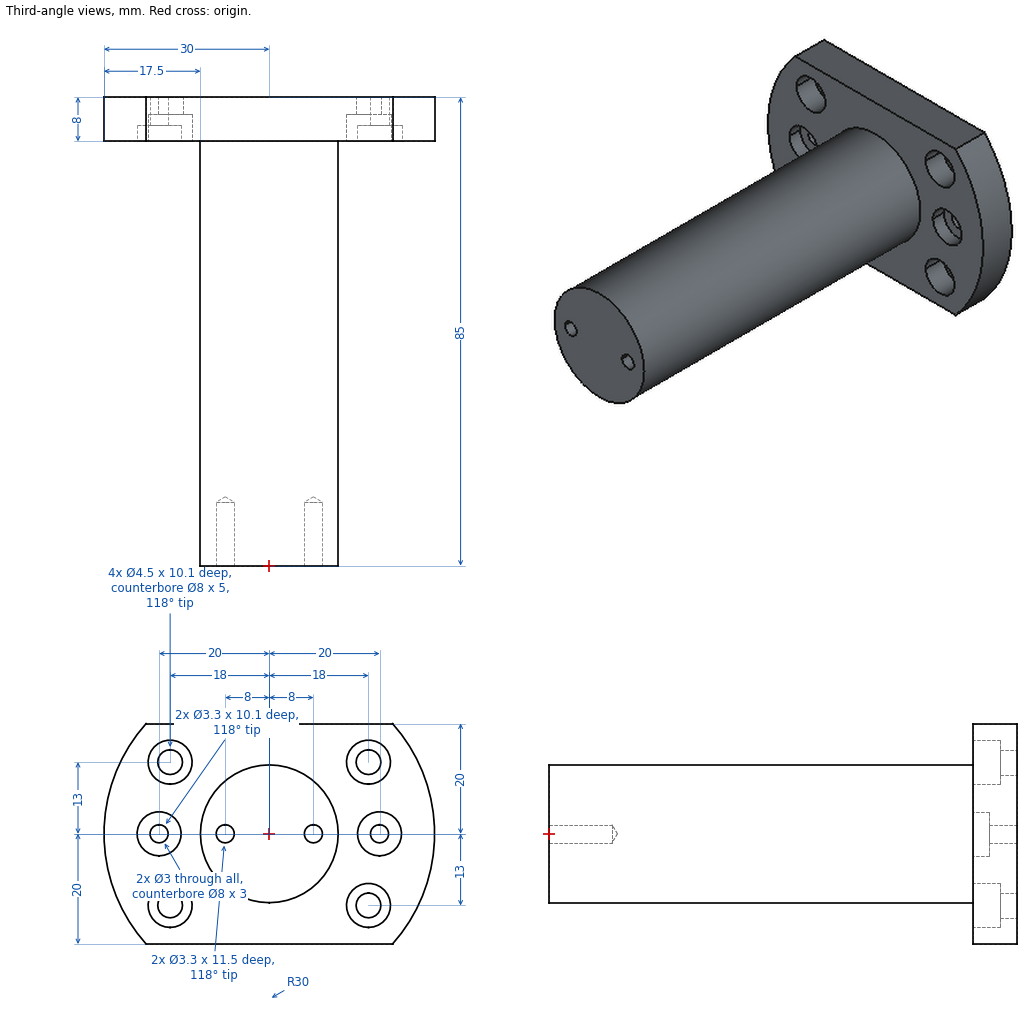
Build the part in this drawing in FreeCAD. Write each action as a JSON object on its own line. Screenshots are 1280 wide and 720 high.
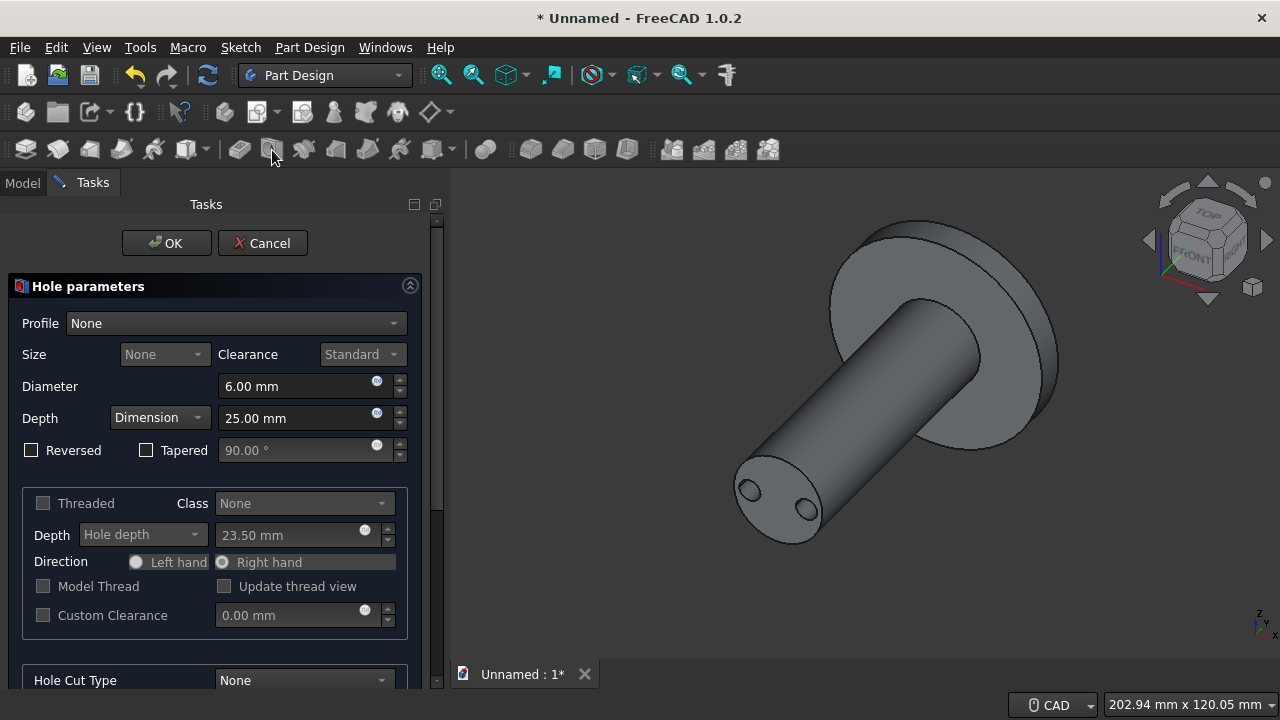
{"action": "triple_click", "coordinate": [305, 386]}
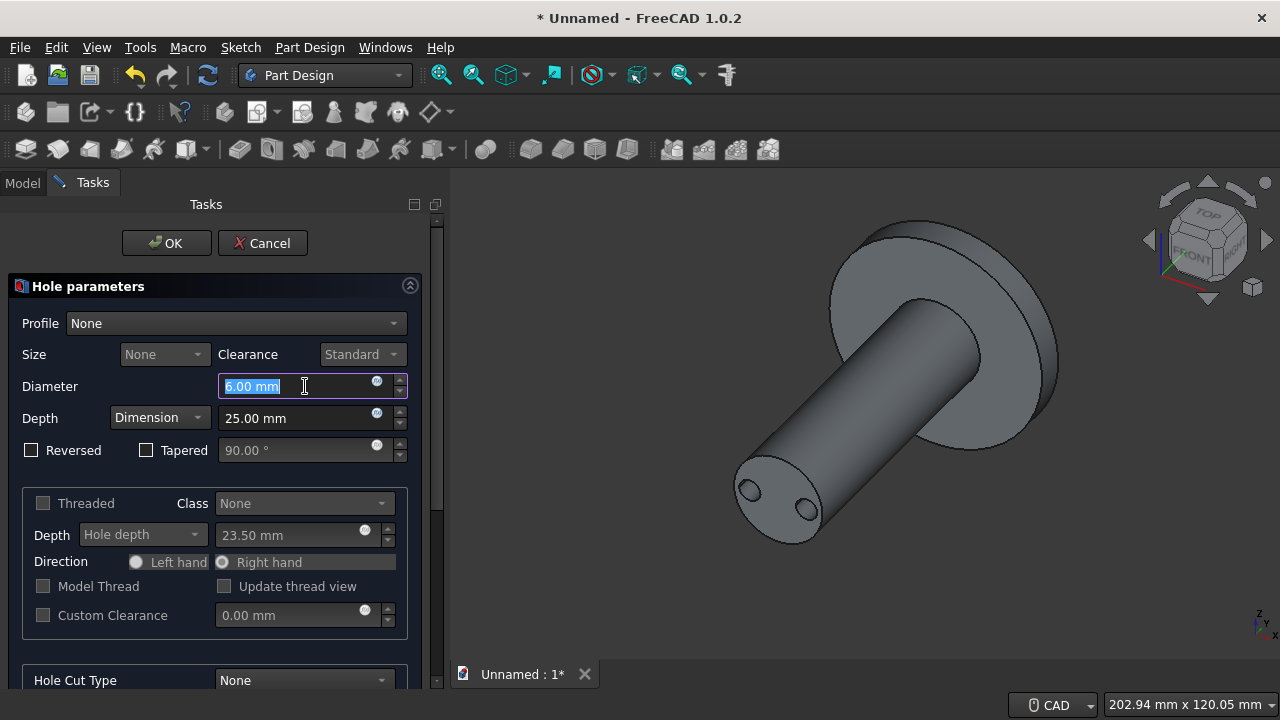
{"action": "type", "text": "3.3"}
{"action": "key", "text": "Tab"}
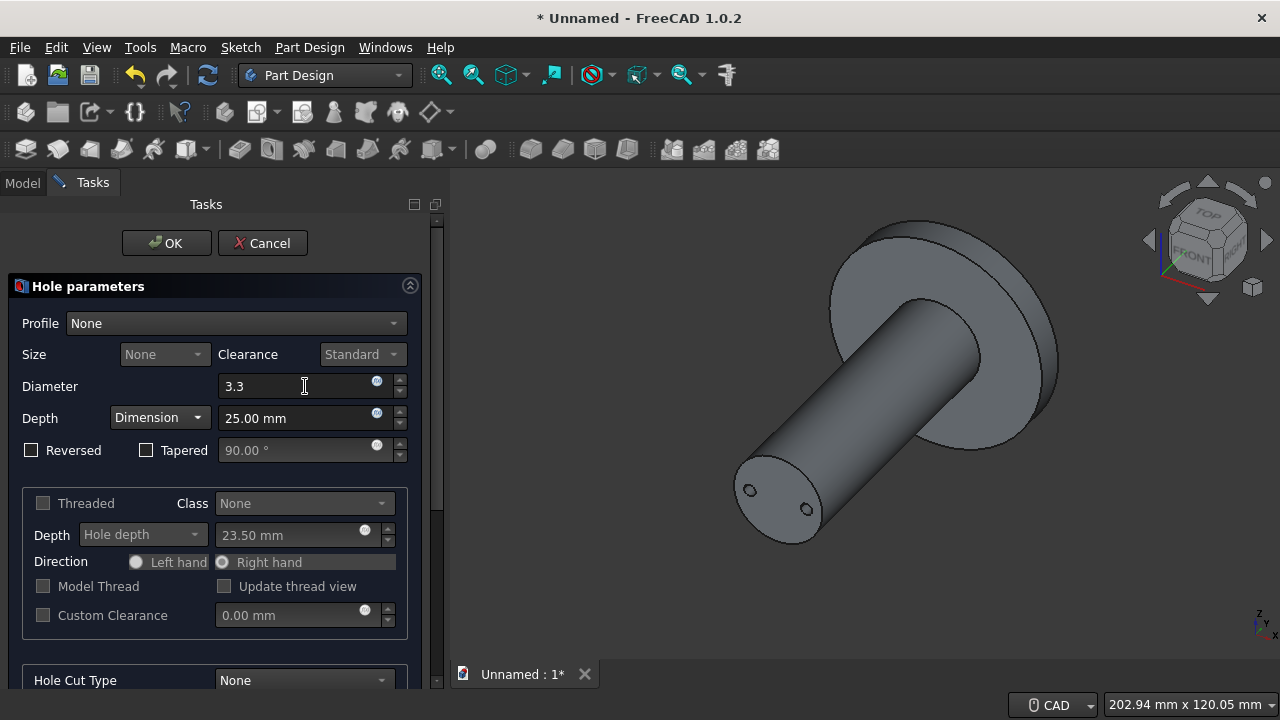
{"action": "triple_click", "coordinate": [305, 418]}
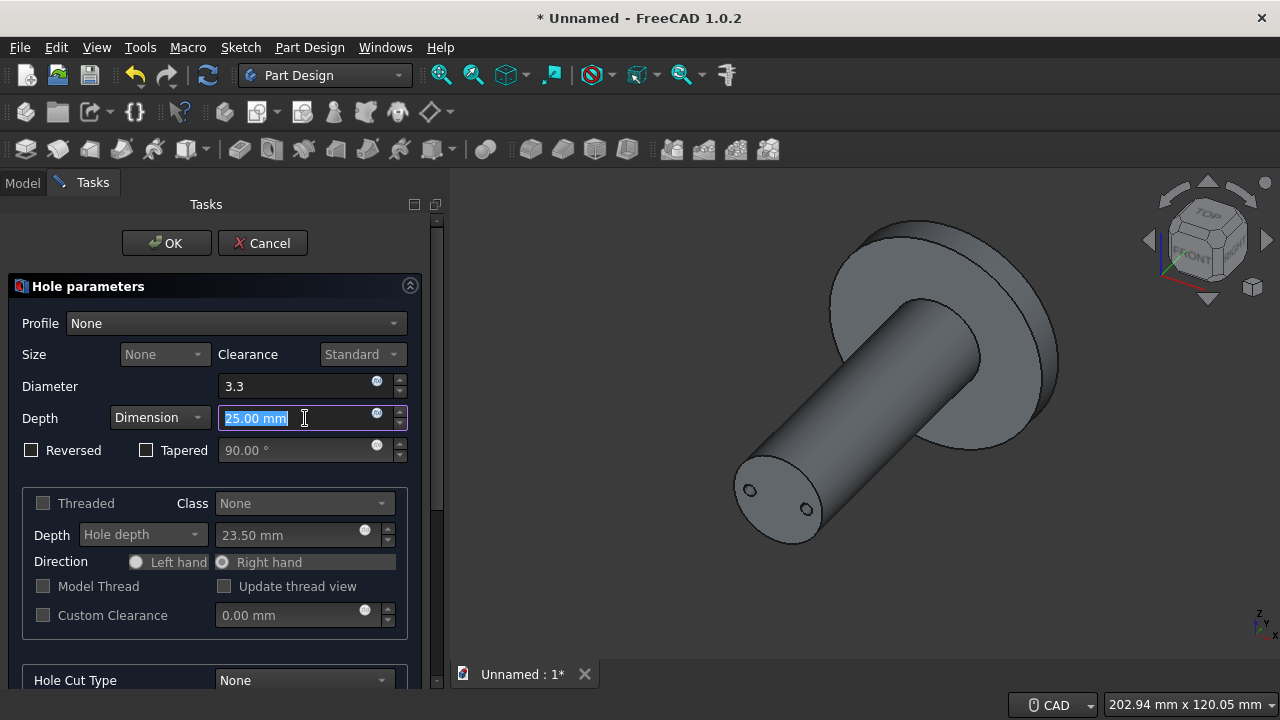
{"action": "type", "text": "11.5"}
{"action": "key", "text": "Tab"}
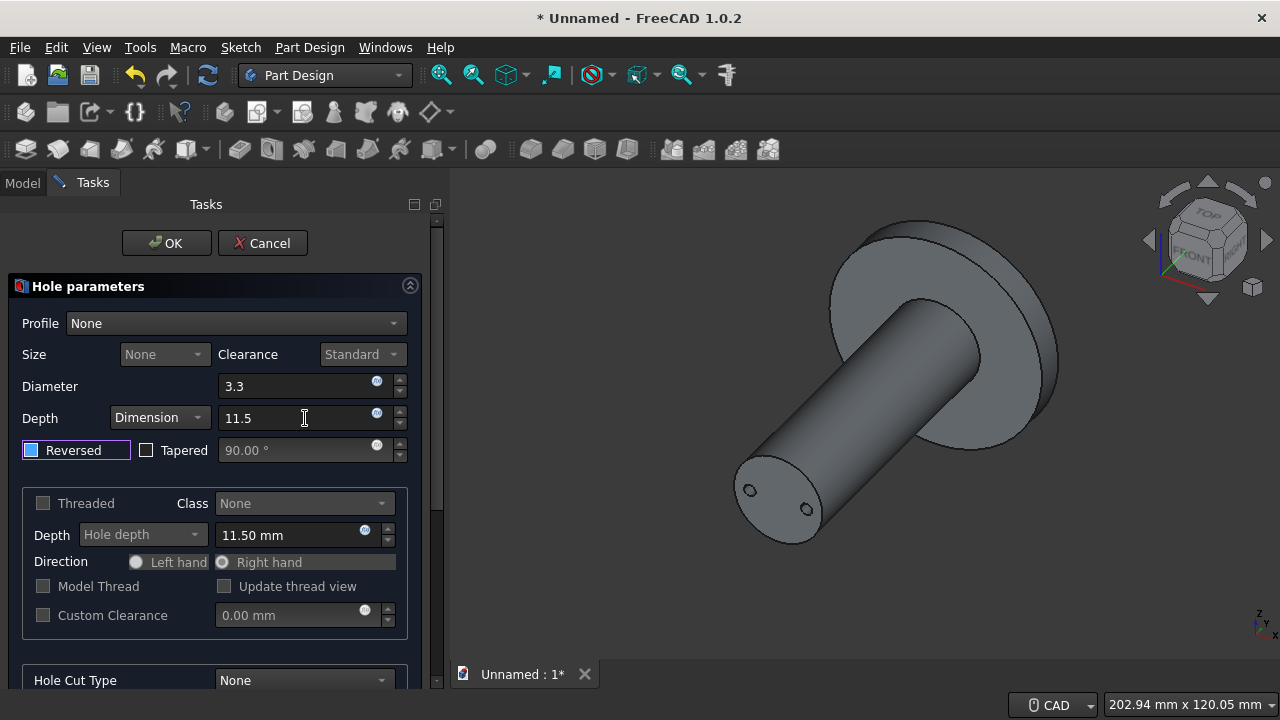
{"action": "left_click", "coordinate": [167, 243]}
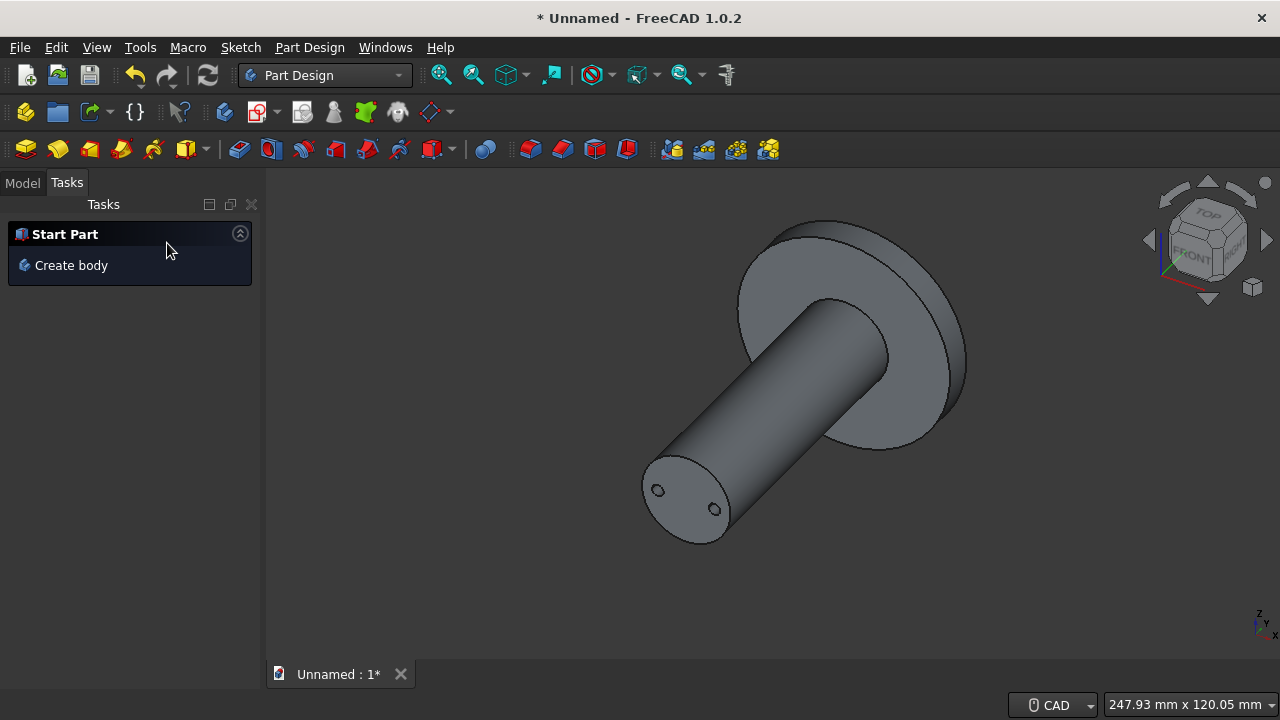
{"action": "key", "text": "4"}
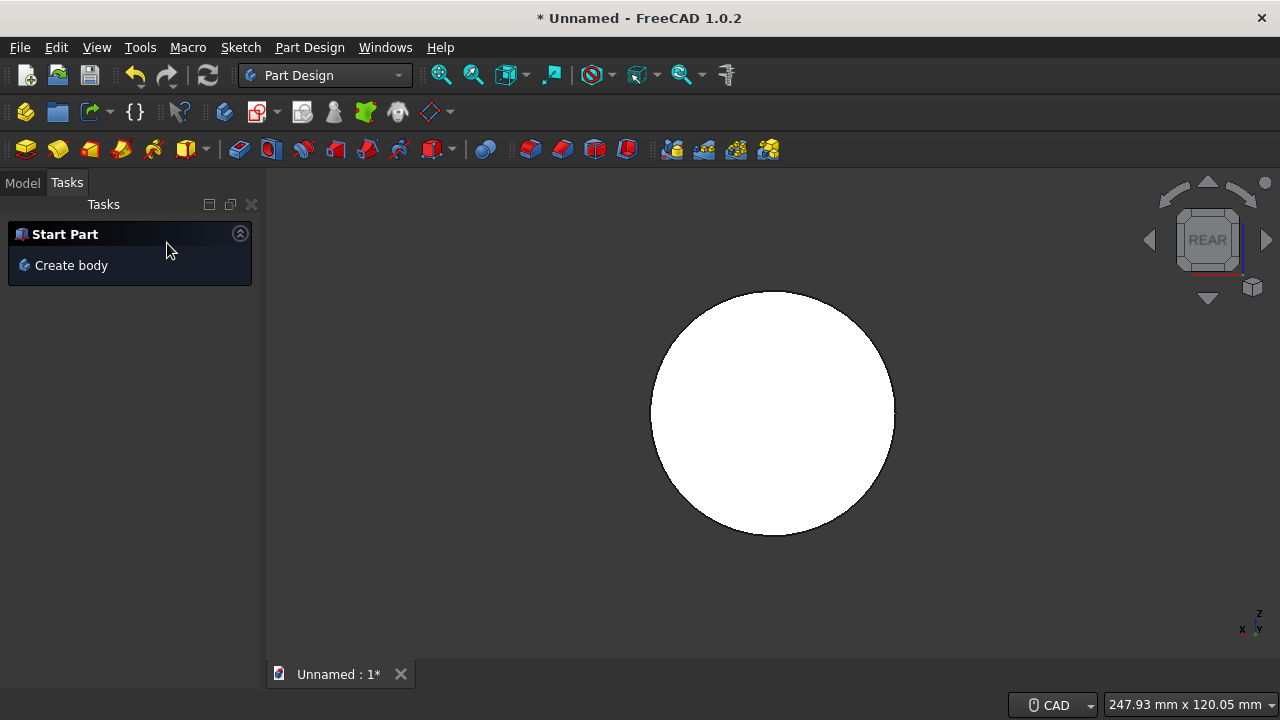
{"action": "left_click", "coordinate": [773, 412]}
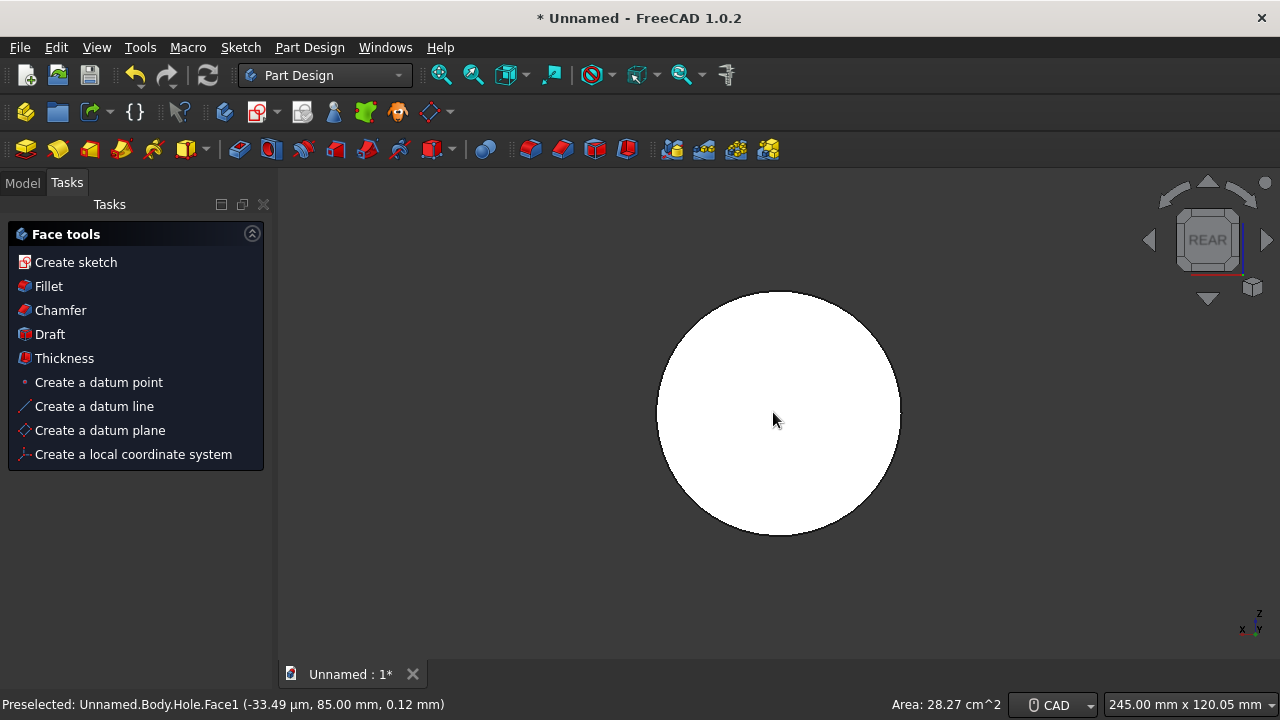
{"action": "left_click", "coordinate": [258, 112]}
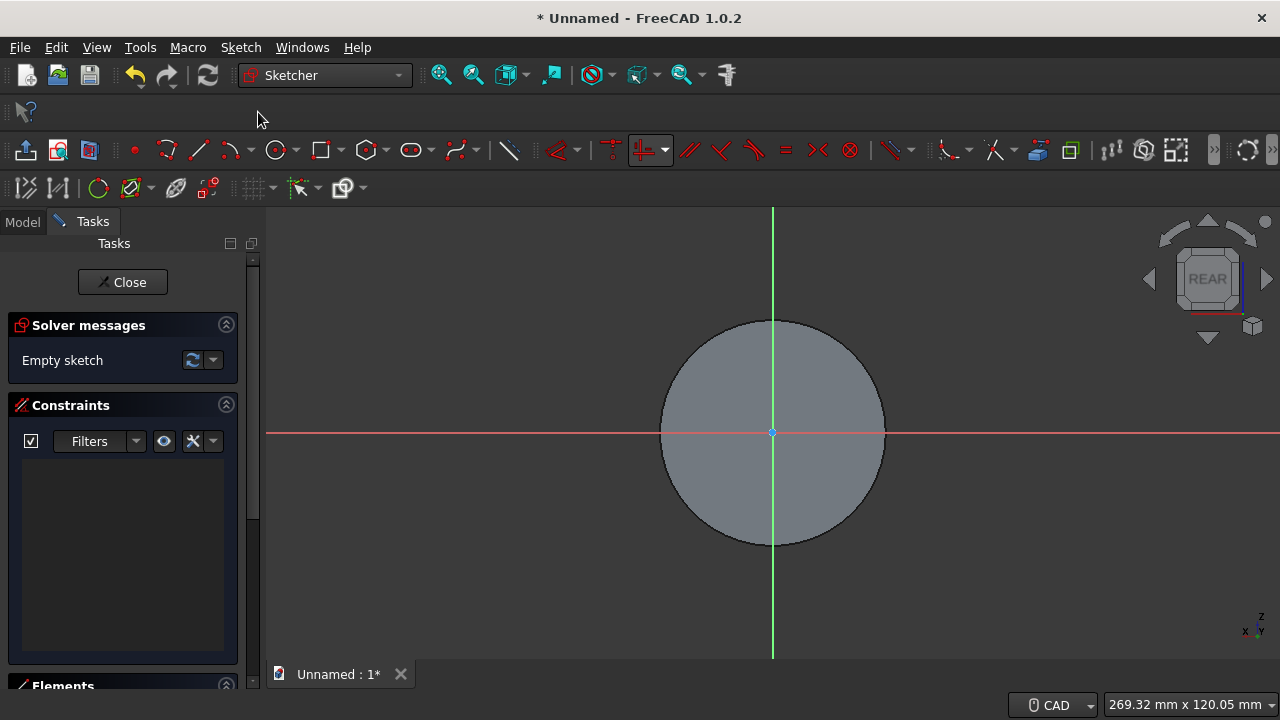
{"action": "scroll", "coordinate": [813, 522], "scroll_direction": "up", "scroll_amount": 5}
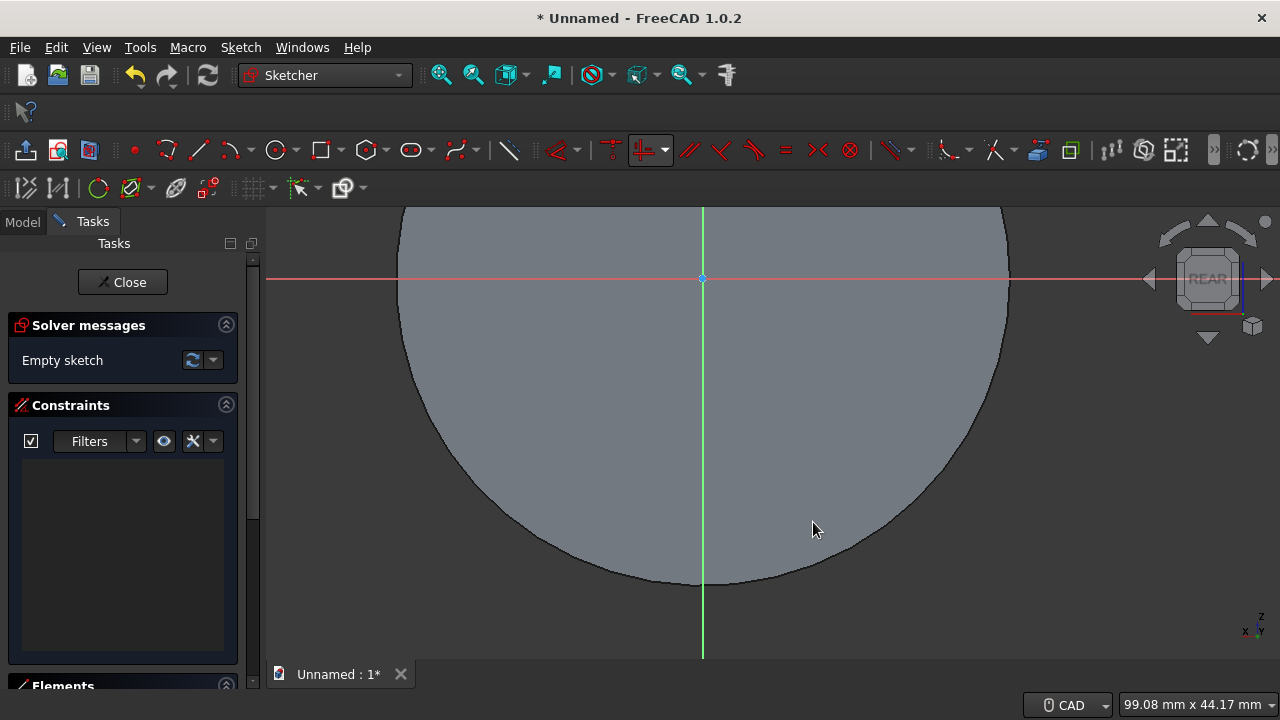
{"action": "left_click", "coordinate": [200, 150]}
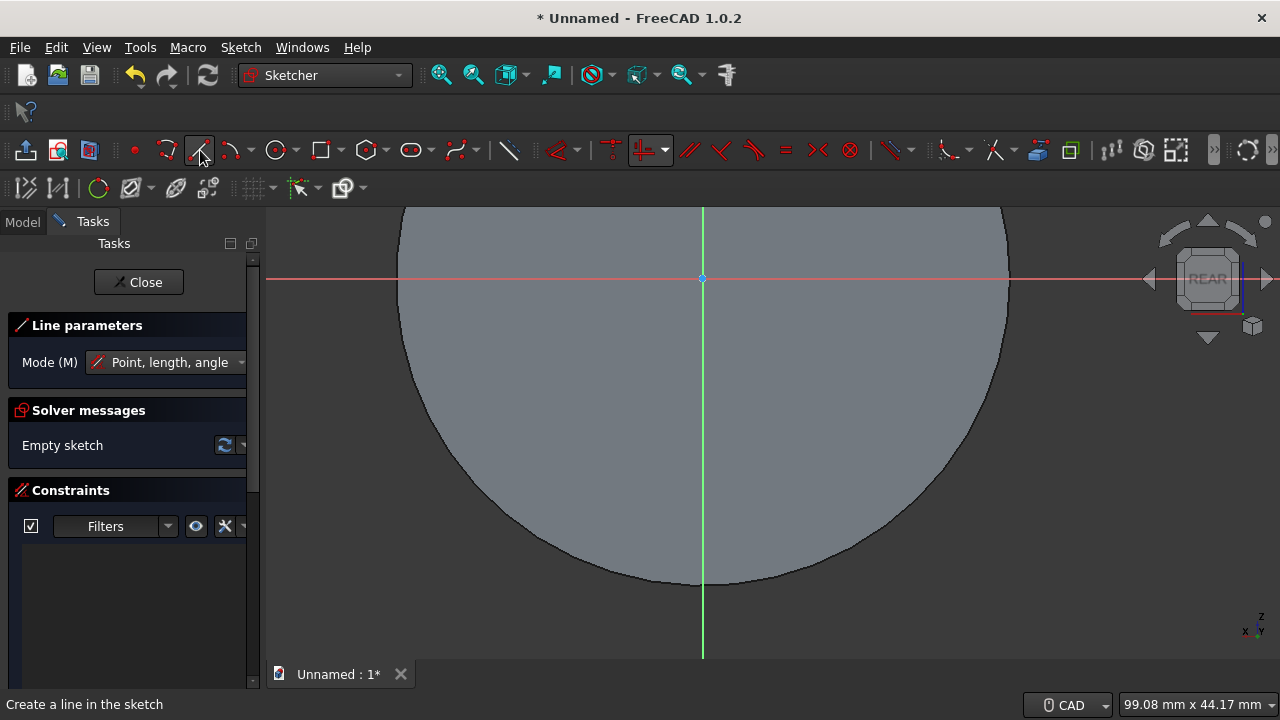
{"action": "left_click", "coordinate": [932, 484]}
{"action": "left_click", "coordinate": [474, 484]}